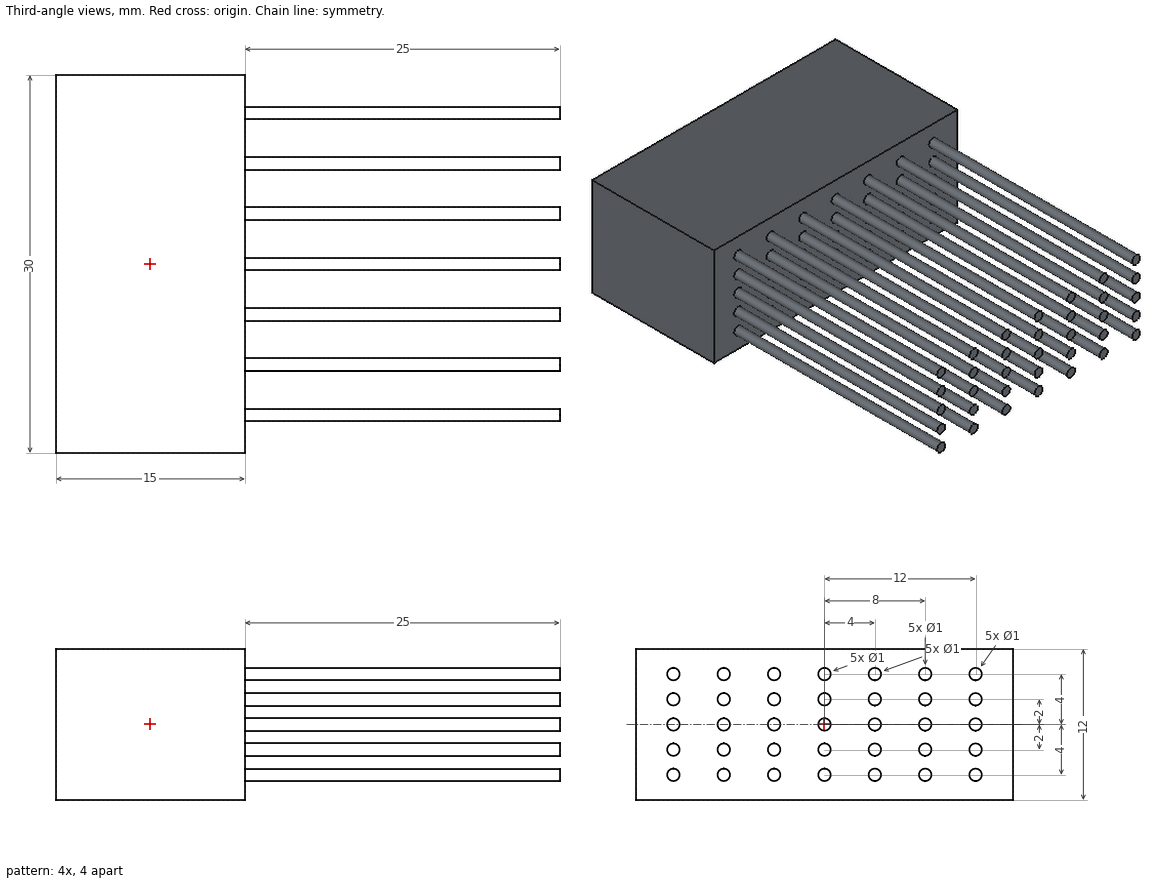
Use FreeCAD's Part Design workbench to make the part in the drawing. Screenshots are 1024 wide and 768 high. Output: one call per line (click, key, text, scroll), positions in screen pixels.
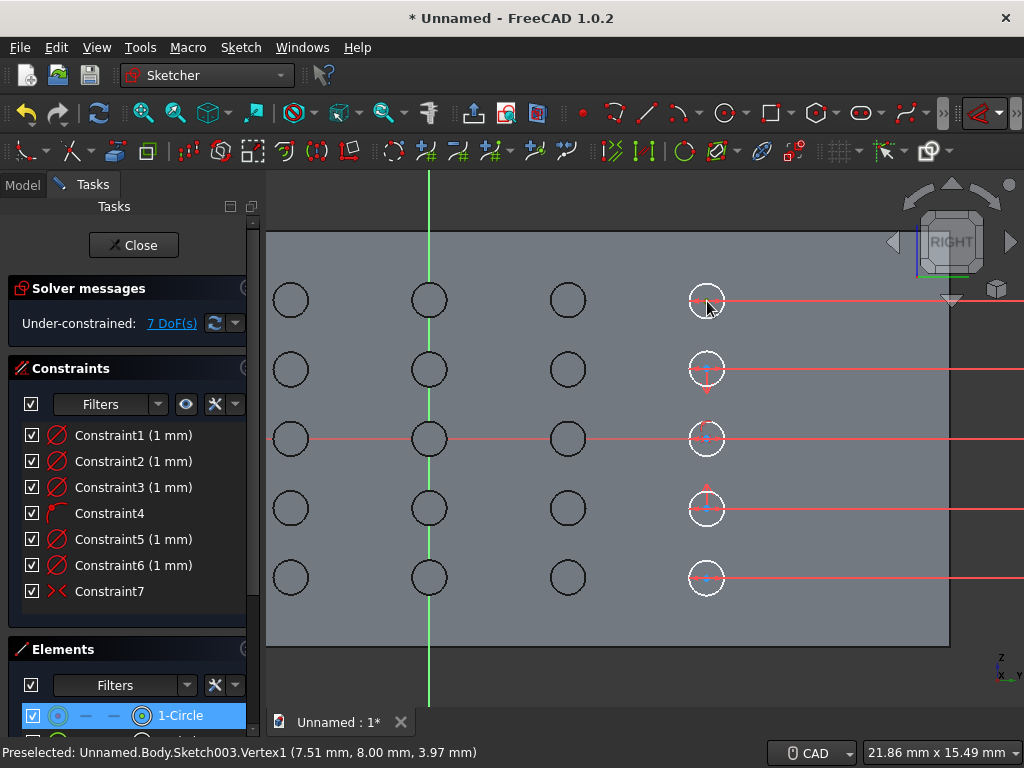
click(707, 578)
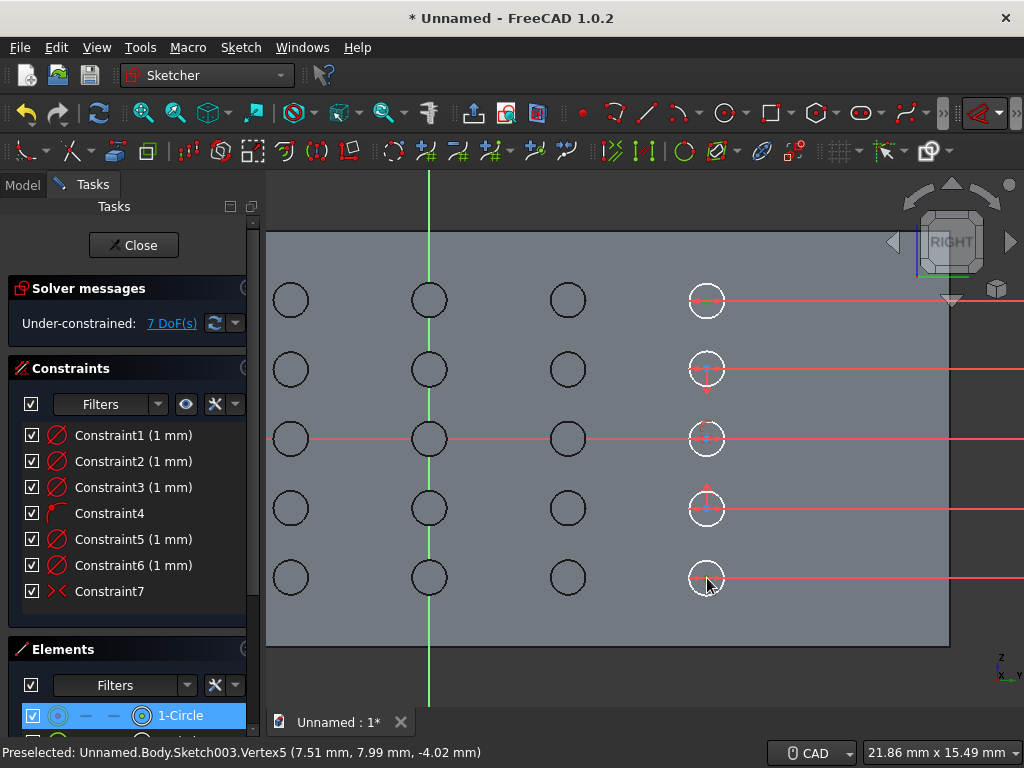
click(334, 439)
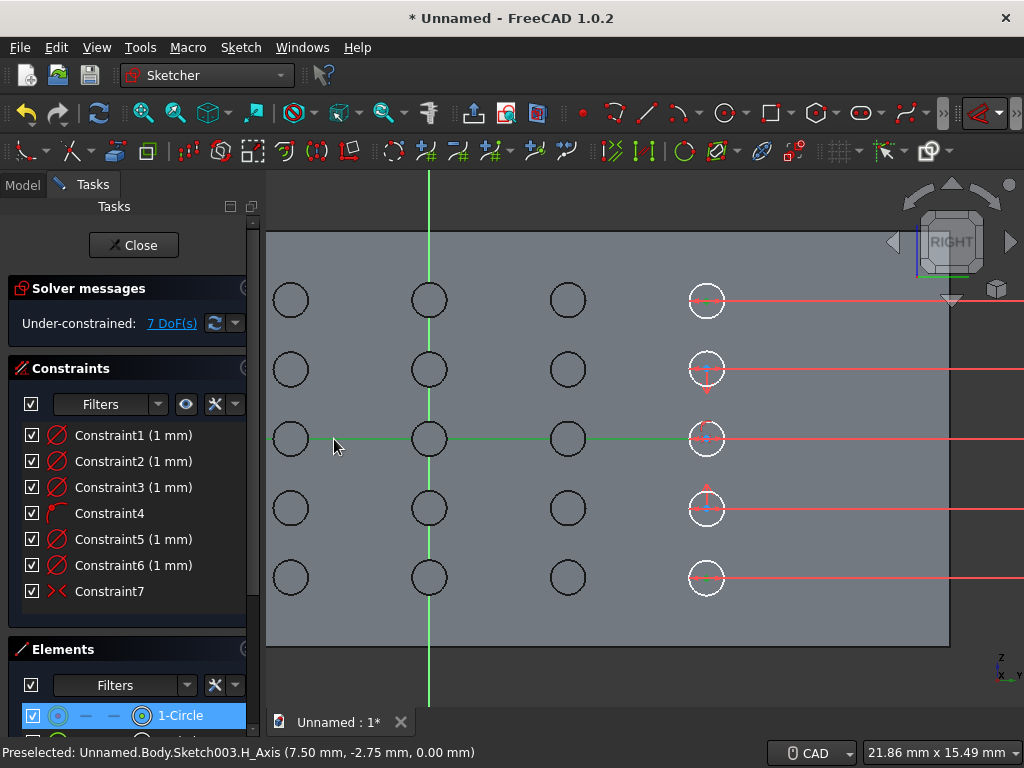
key(s)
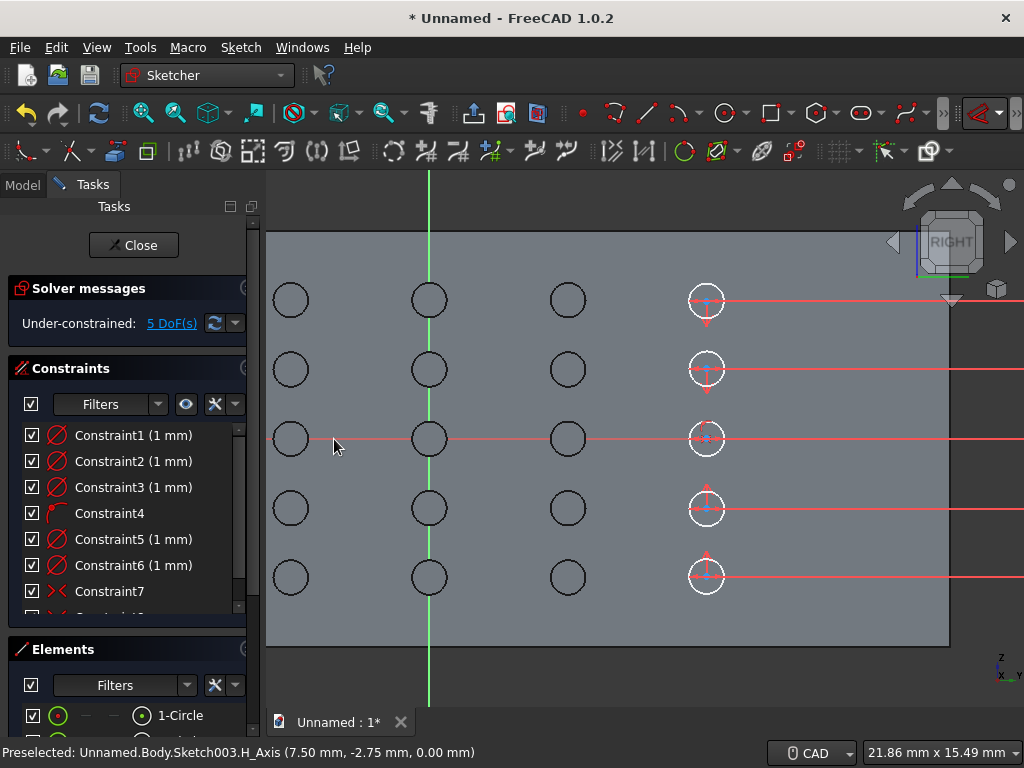
click(707, 301)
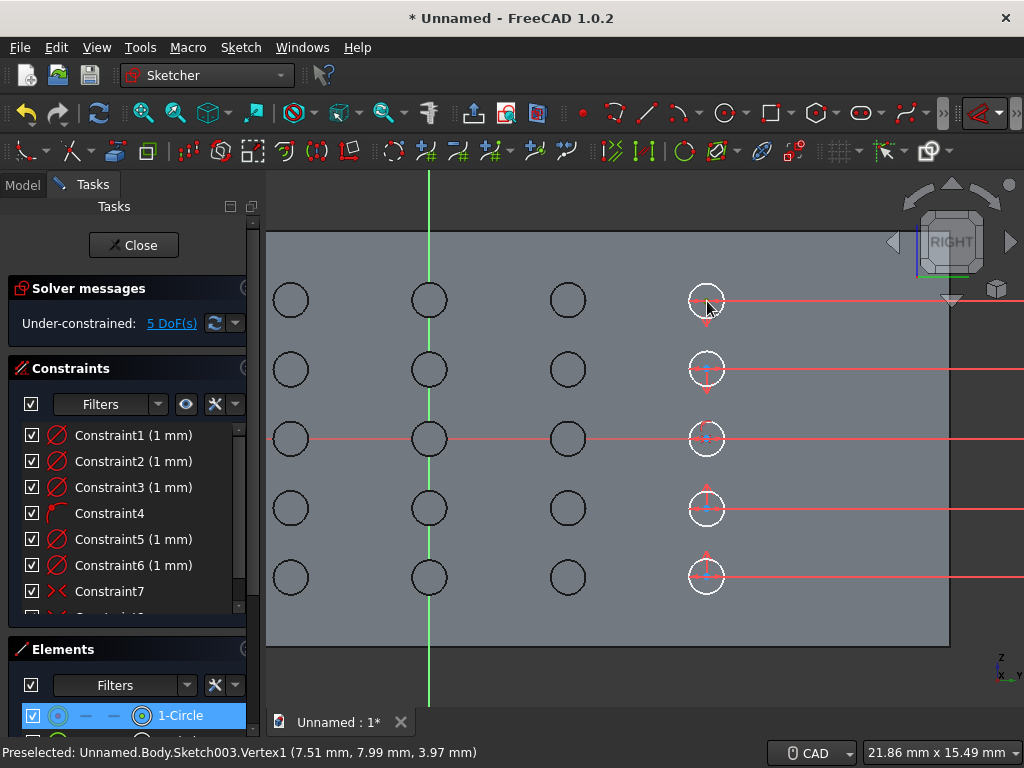
key(l)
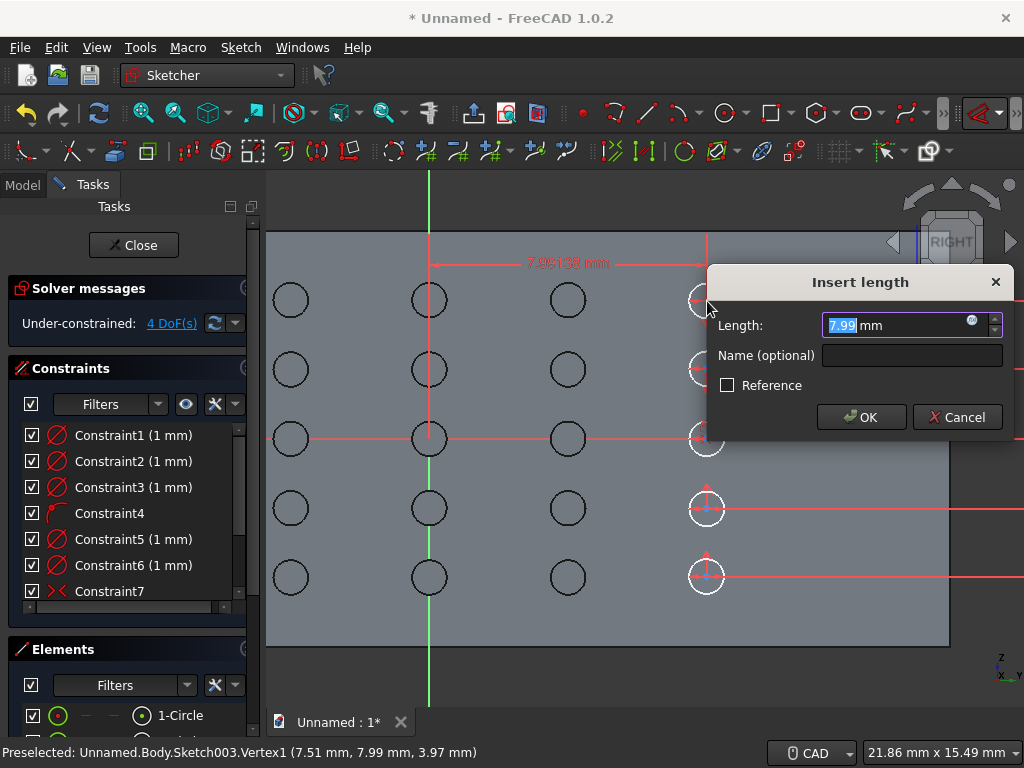
text(8)
key(Return)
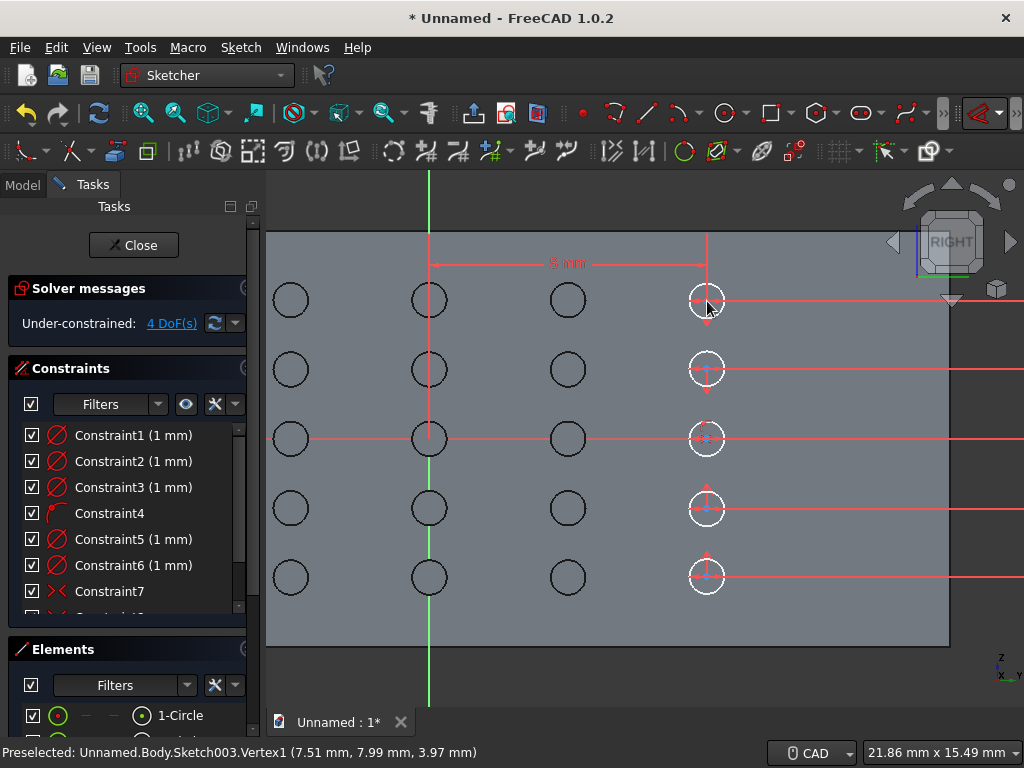
click(707, 301)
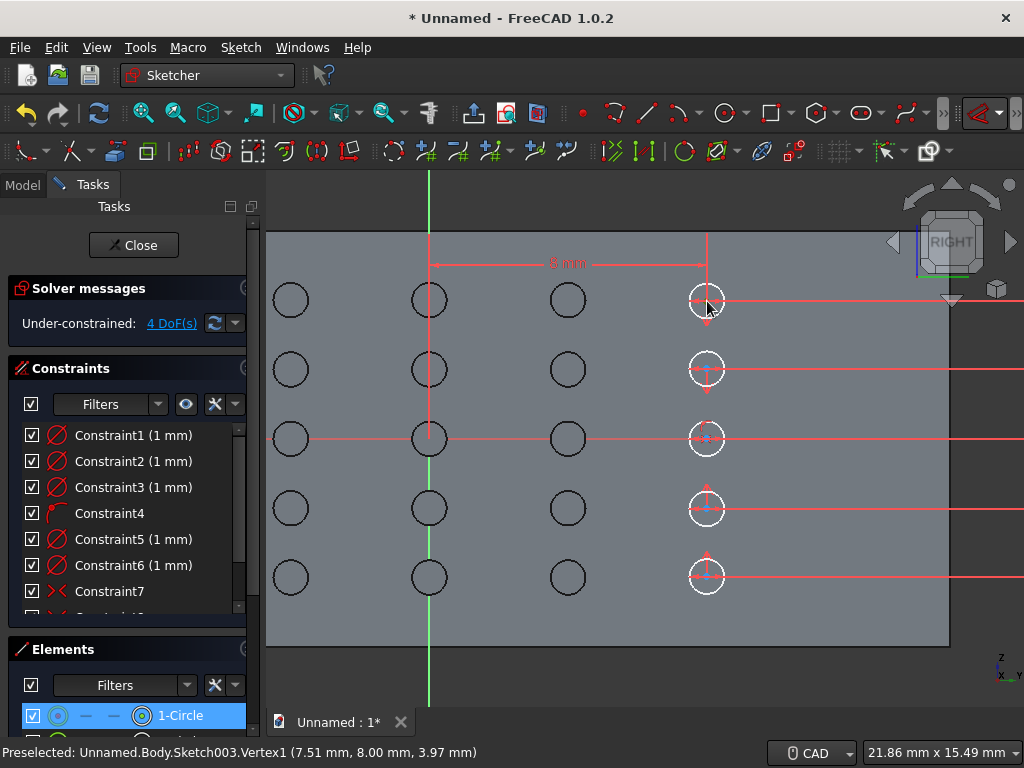
key(i)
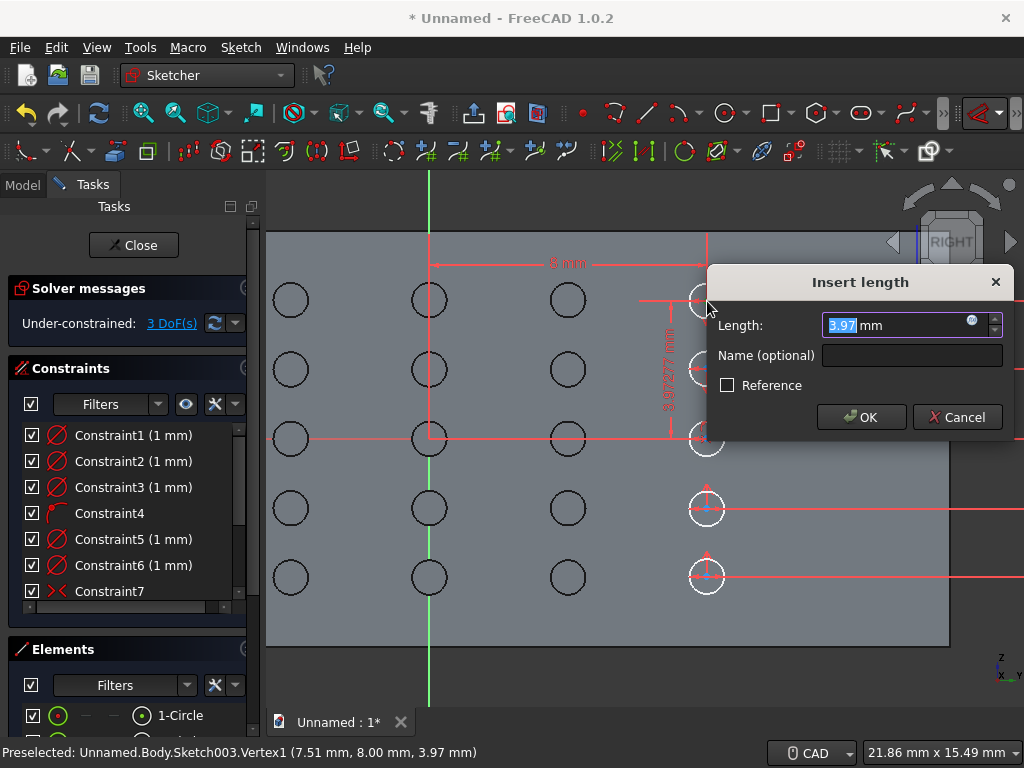
text(4)
key(Return)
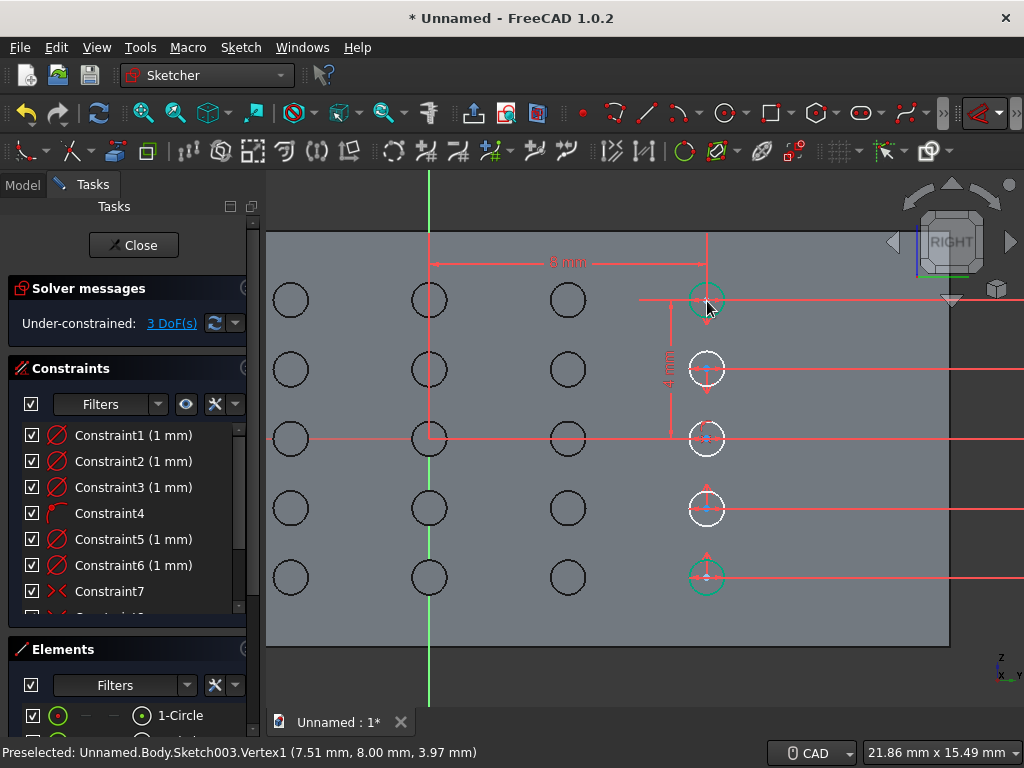
click(707, 369)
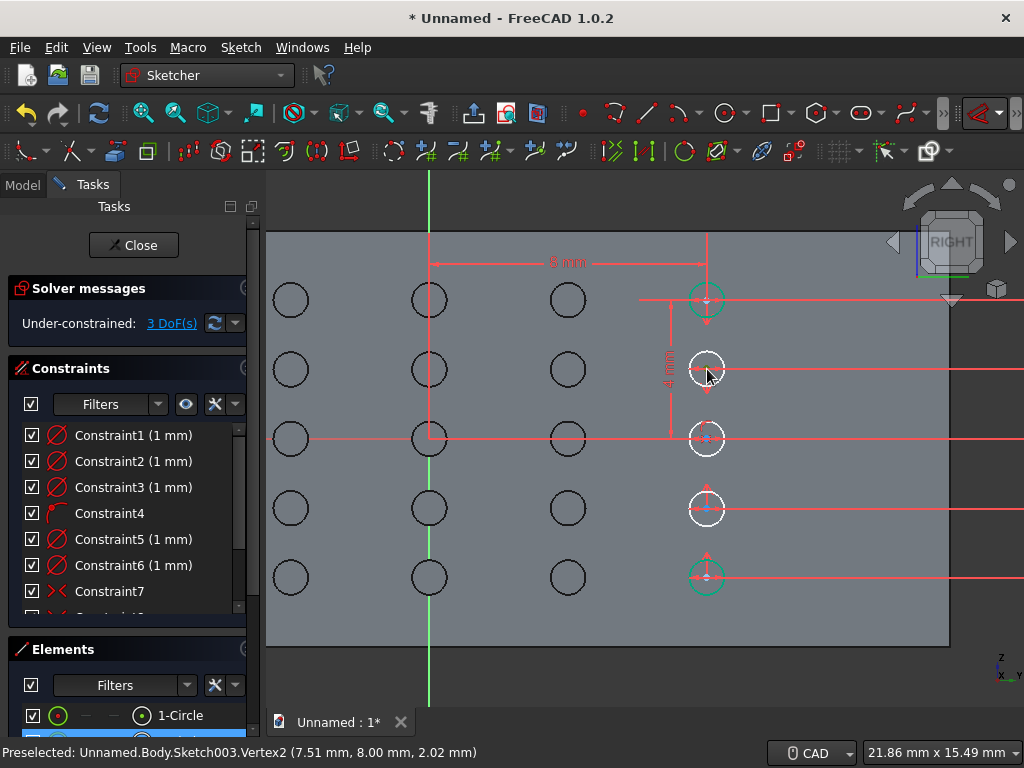
key(l)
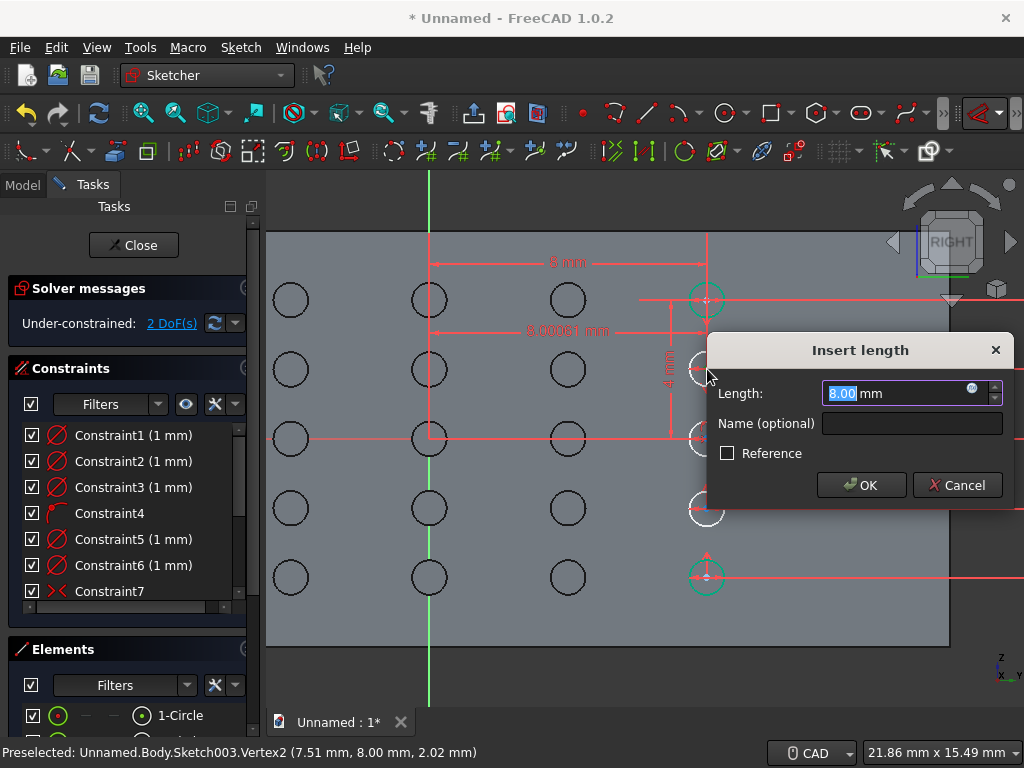
text(8)
key(Return)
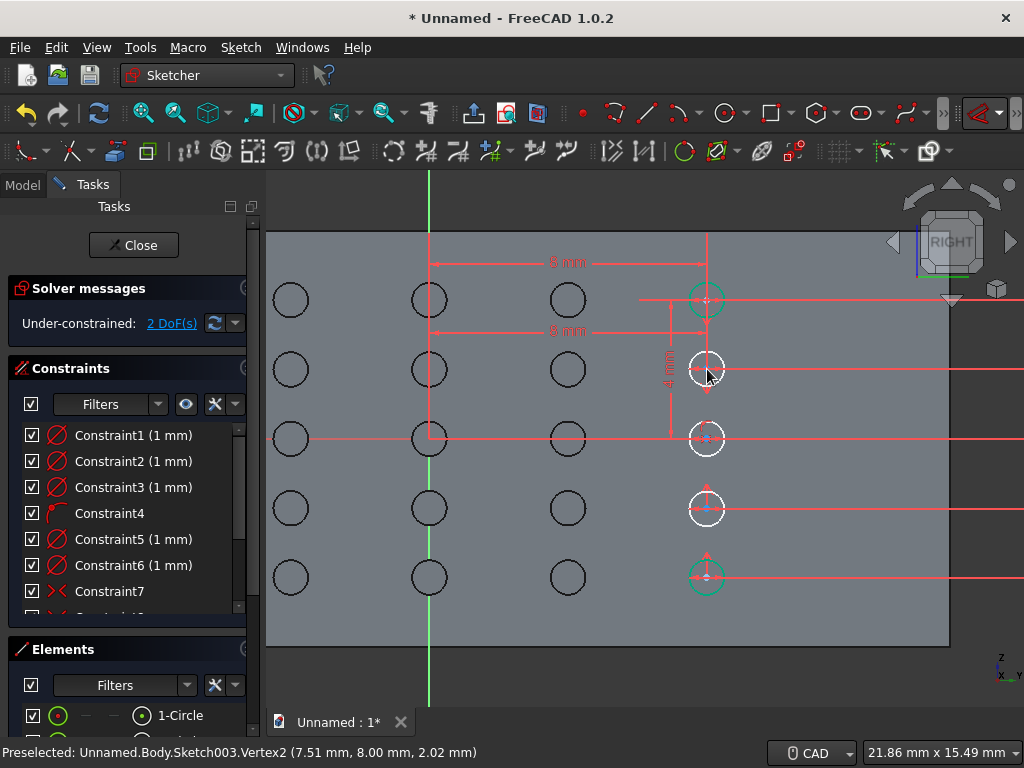
click(707, 369)